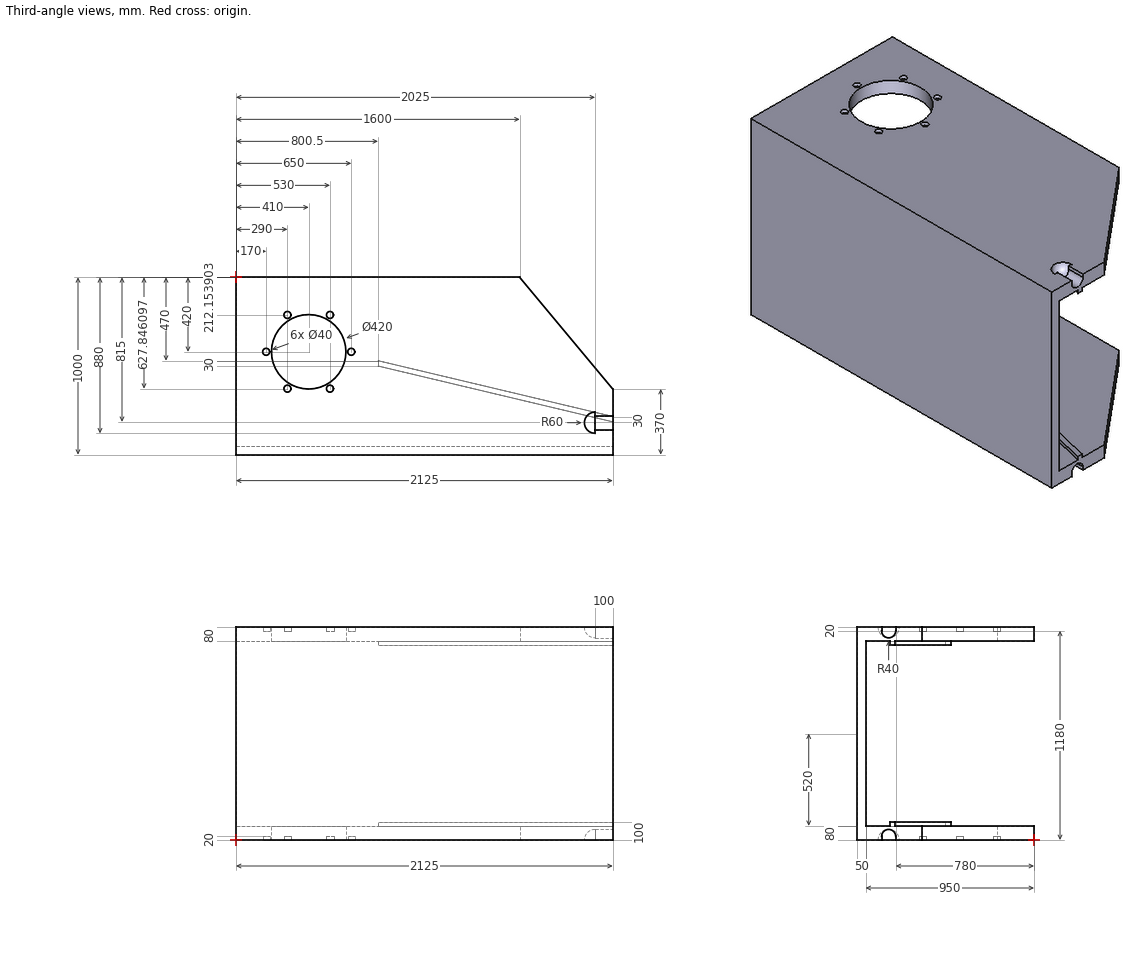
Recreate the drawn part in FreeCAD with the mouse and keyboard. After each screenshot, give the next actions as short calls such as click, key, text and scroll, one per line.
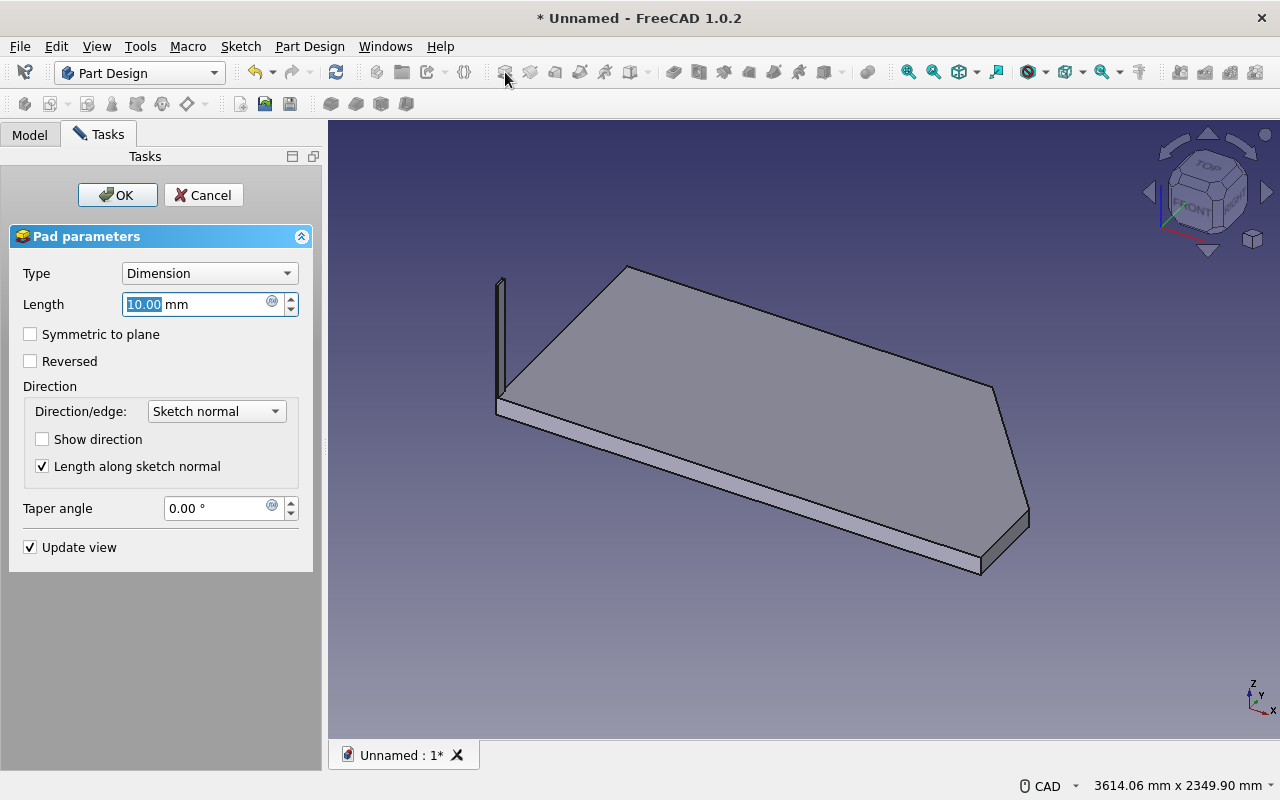
text(2125)
key(Tab)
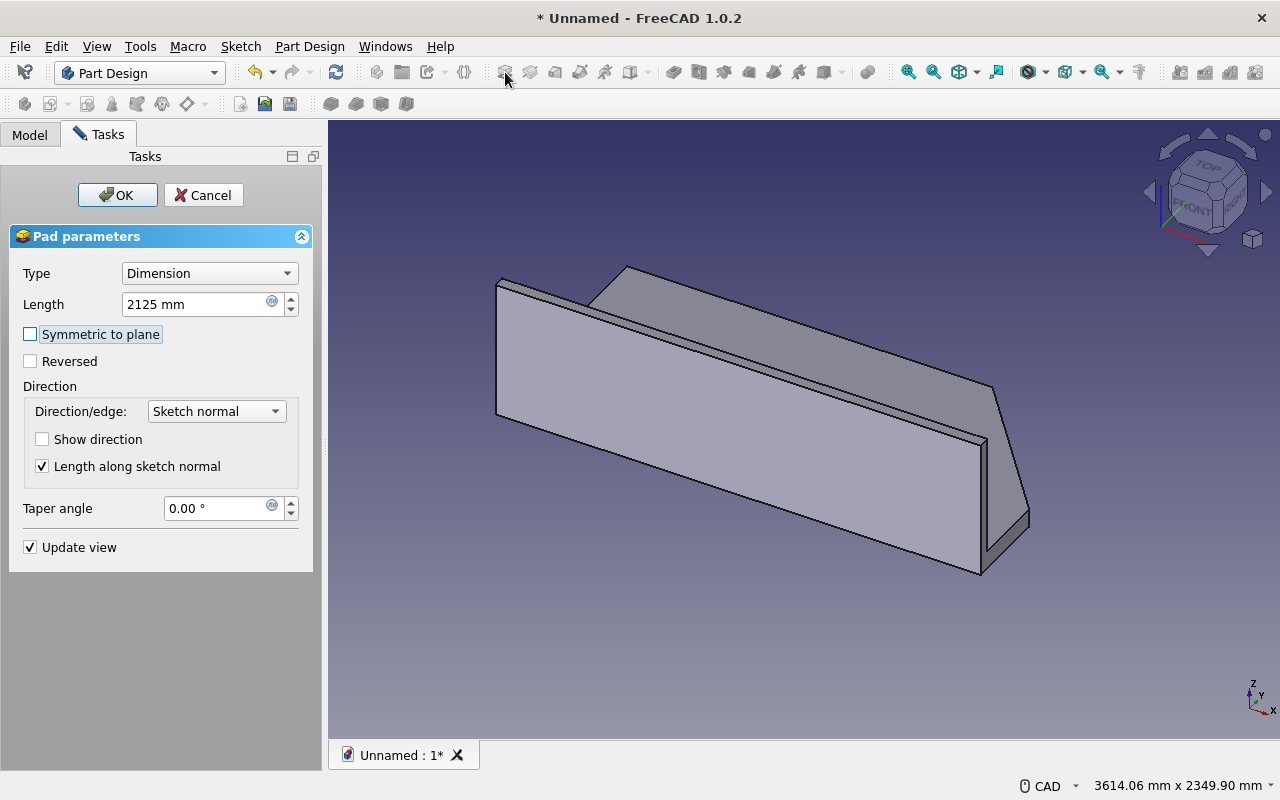
click(118, 195)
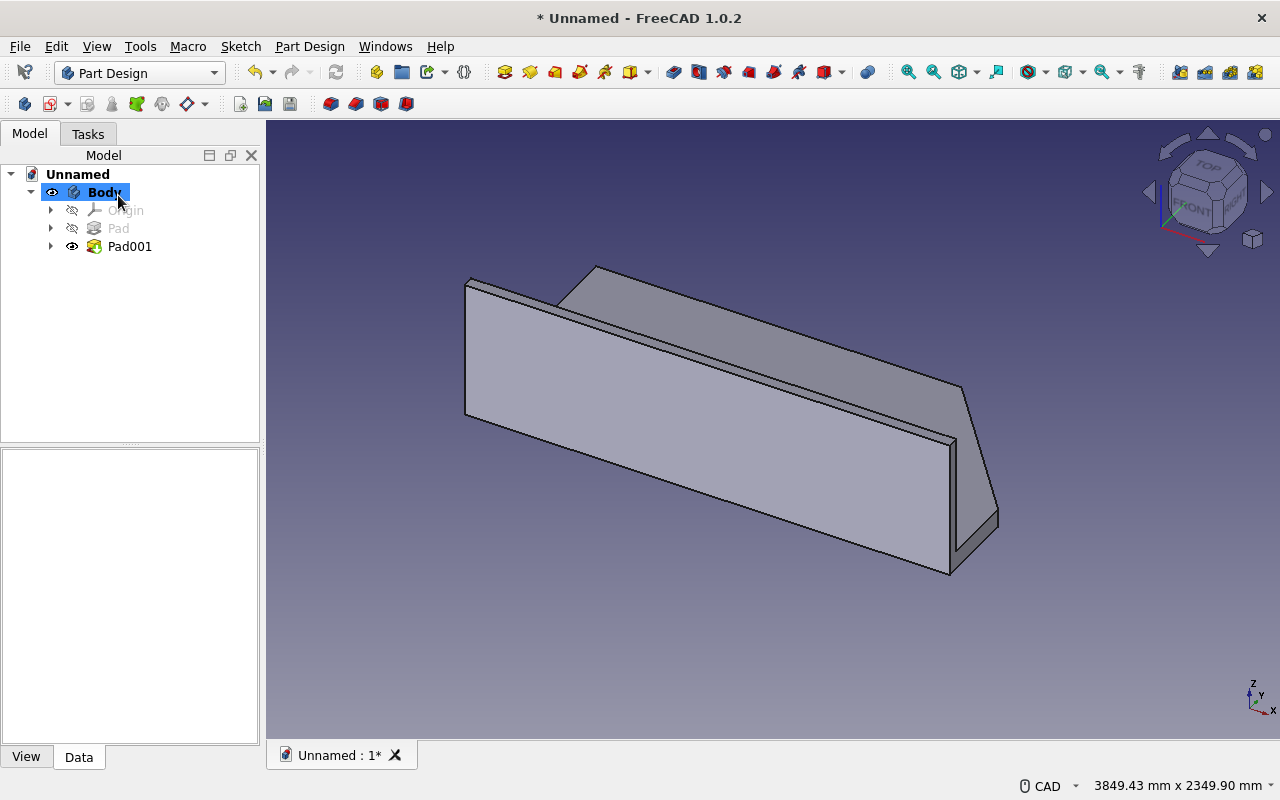
click(51, 210)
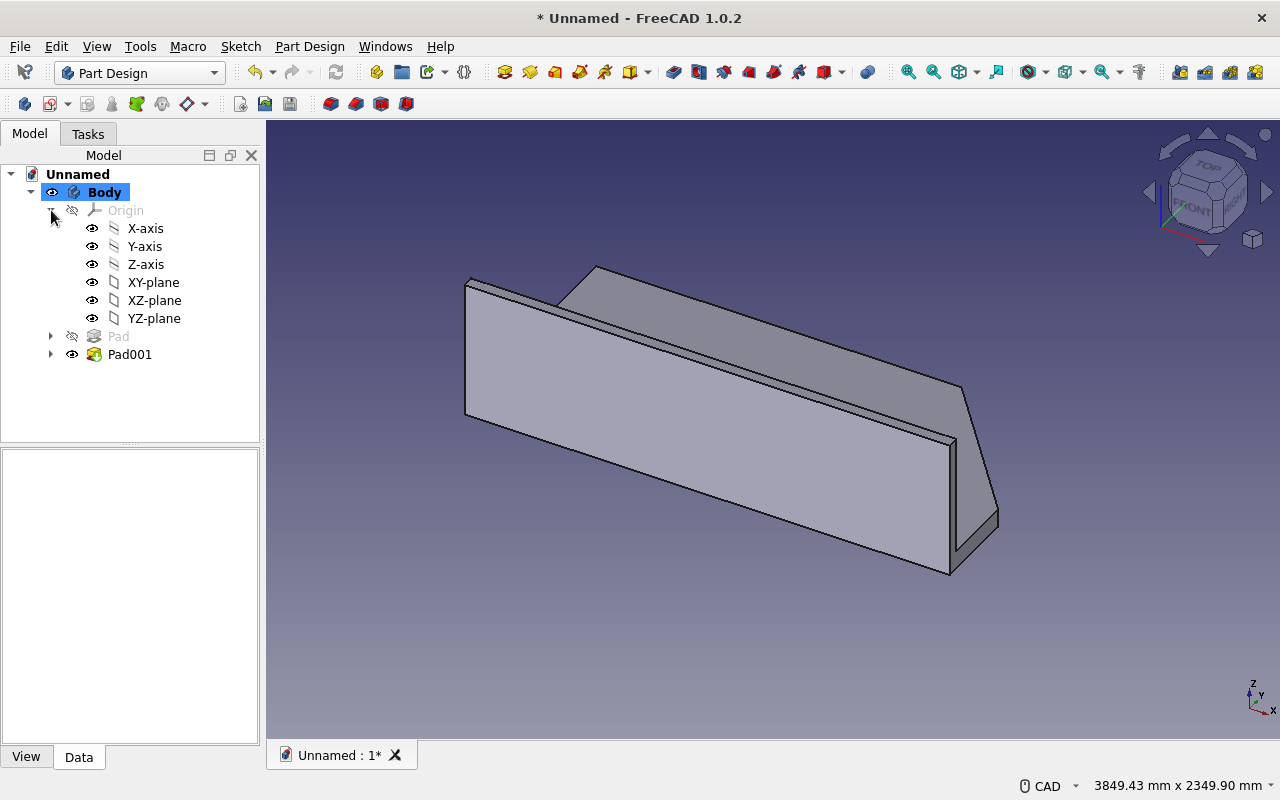
click(137, 282)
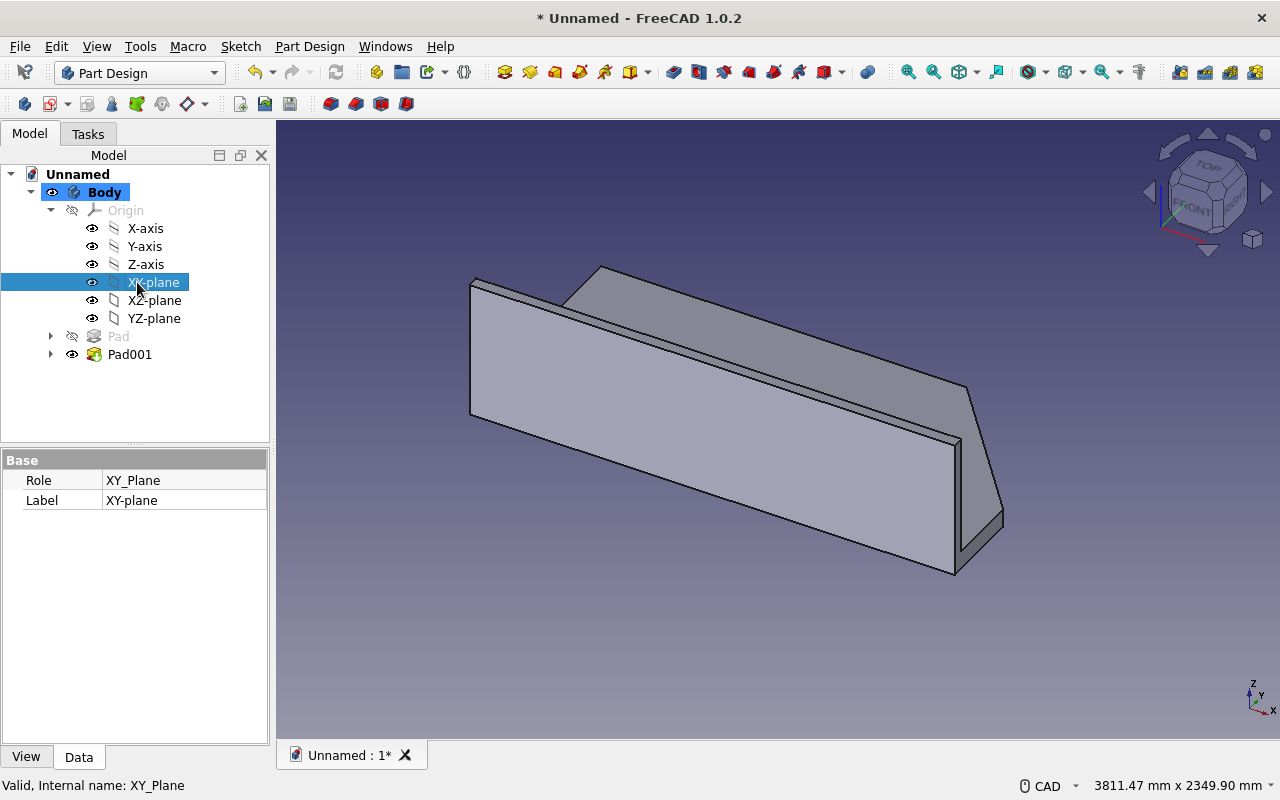
click(186, 104)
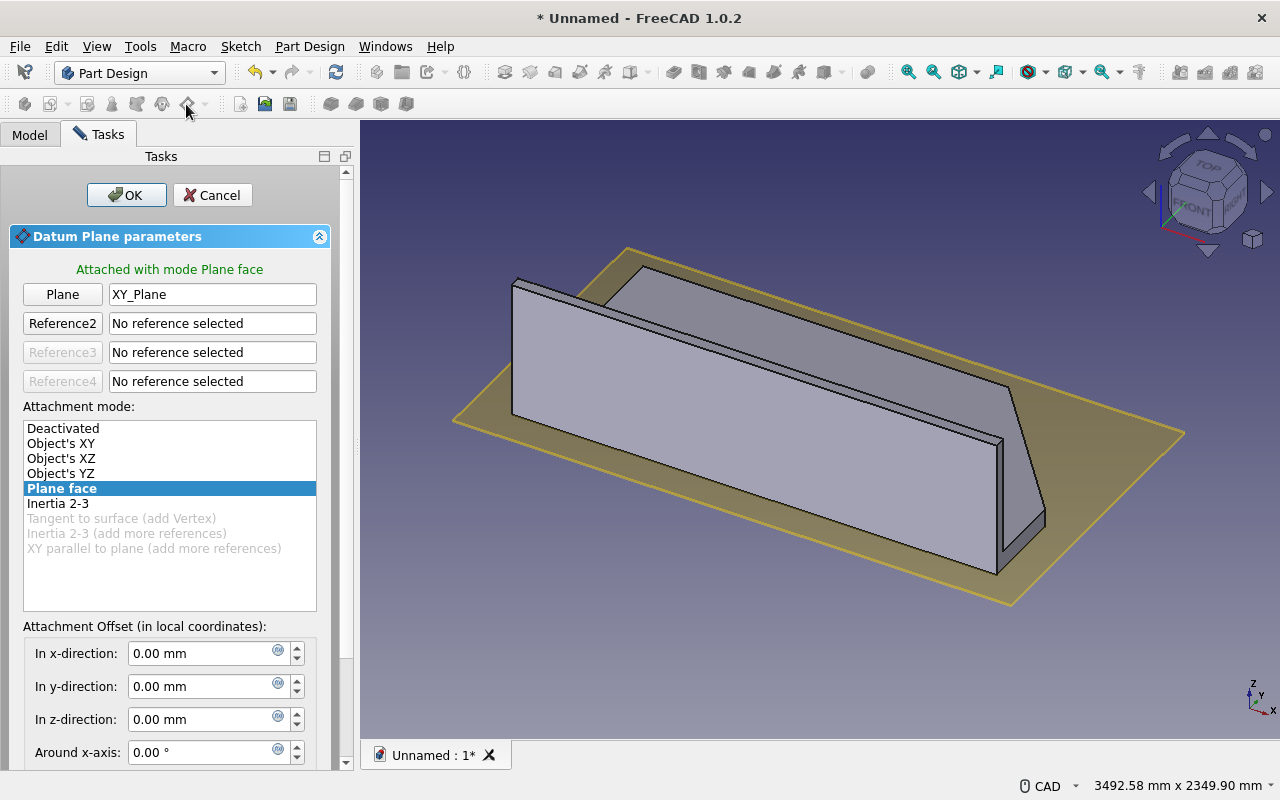
triple_click(210, 720)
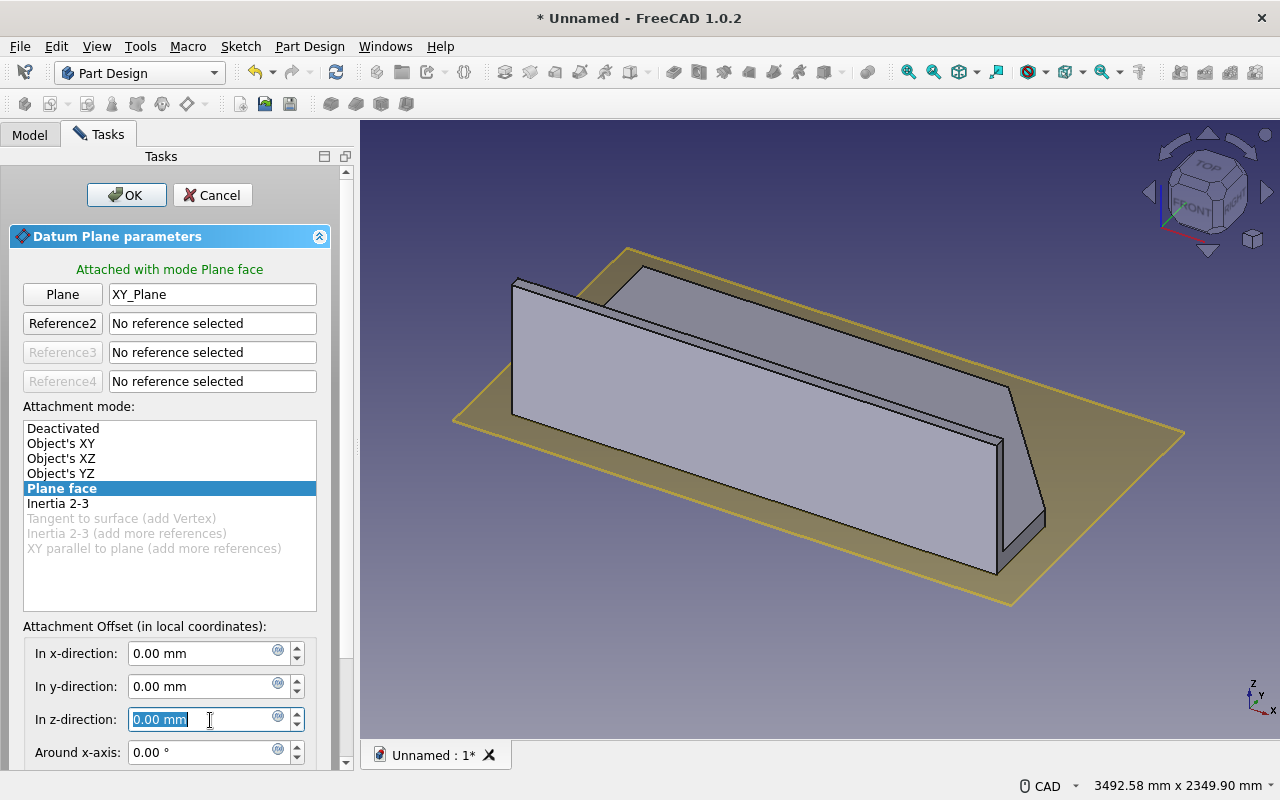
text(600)
key(Tab)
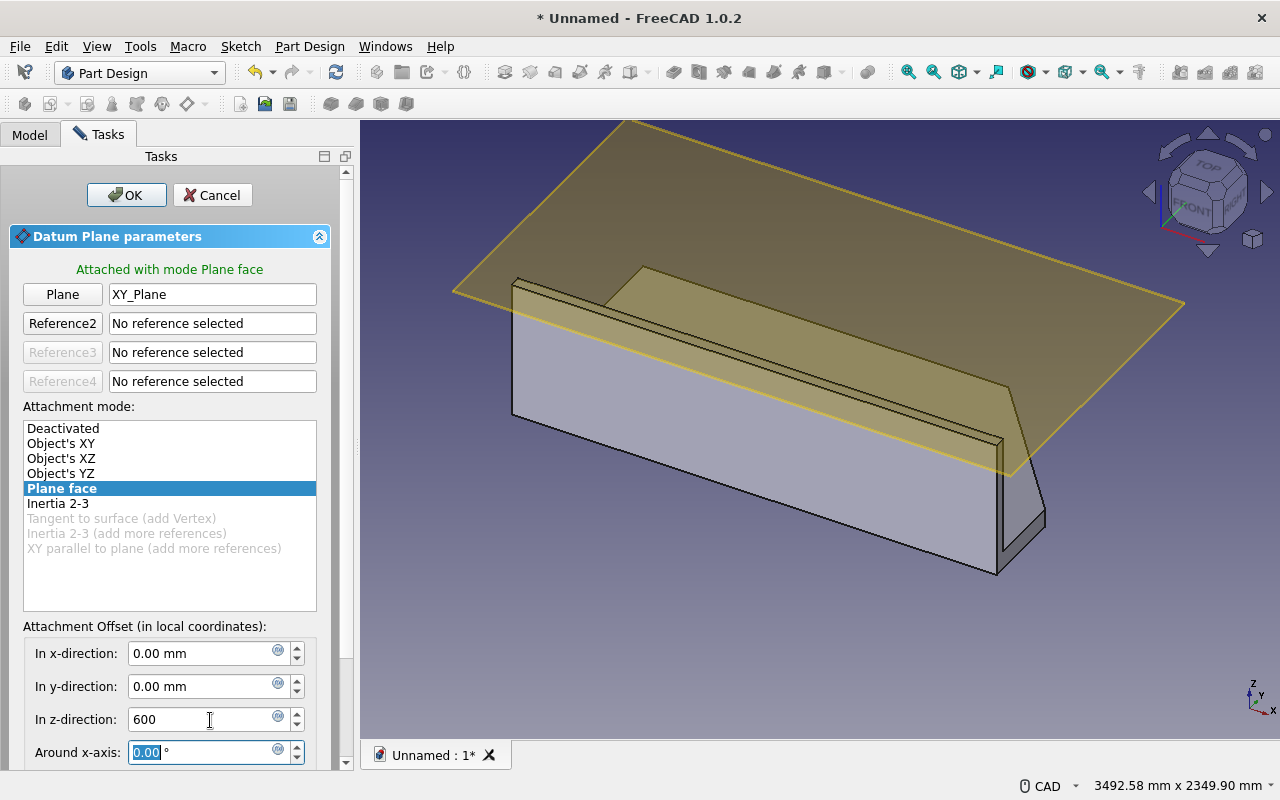
click(127, 195)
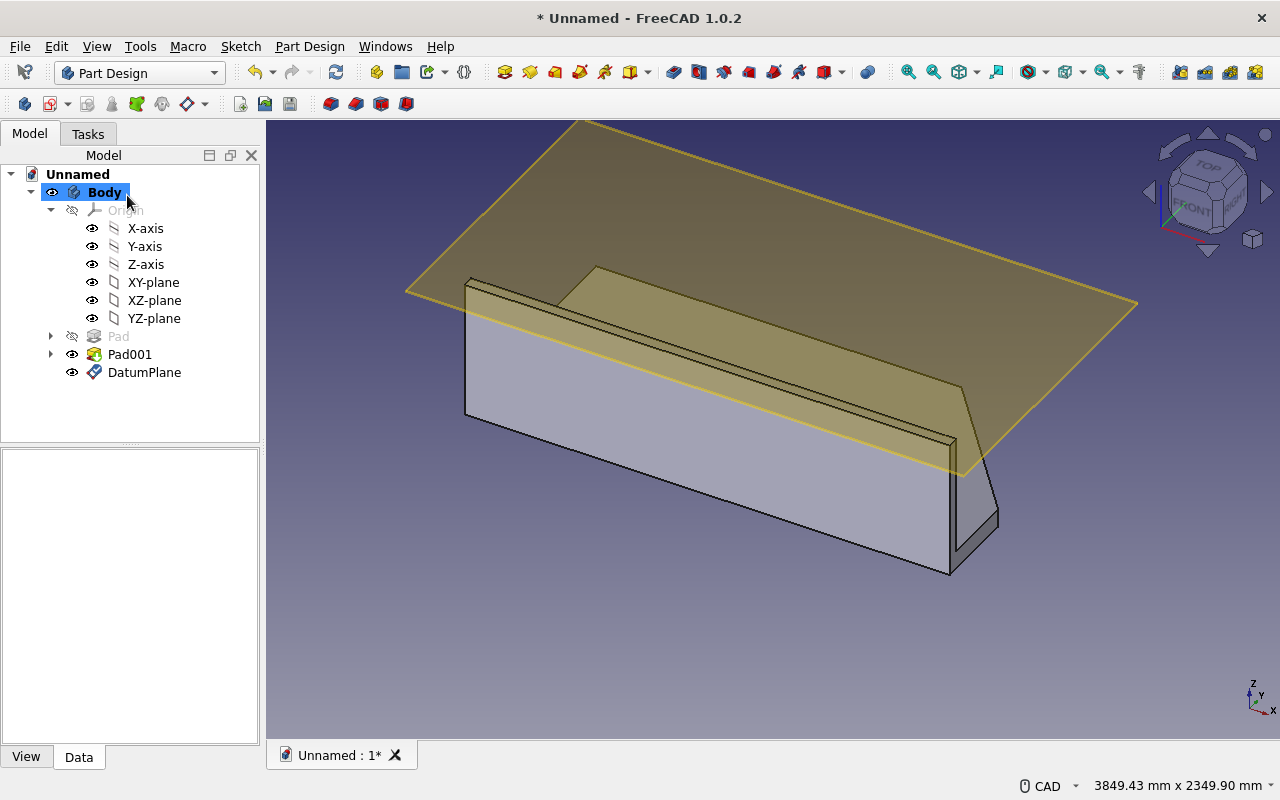
click(117, 354)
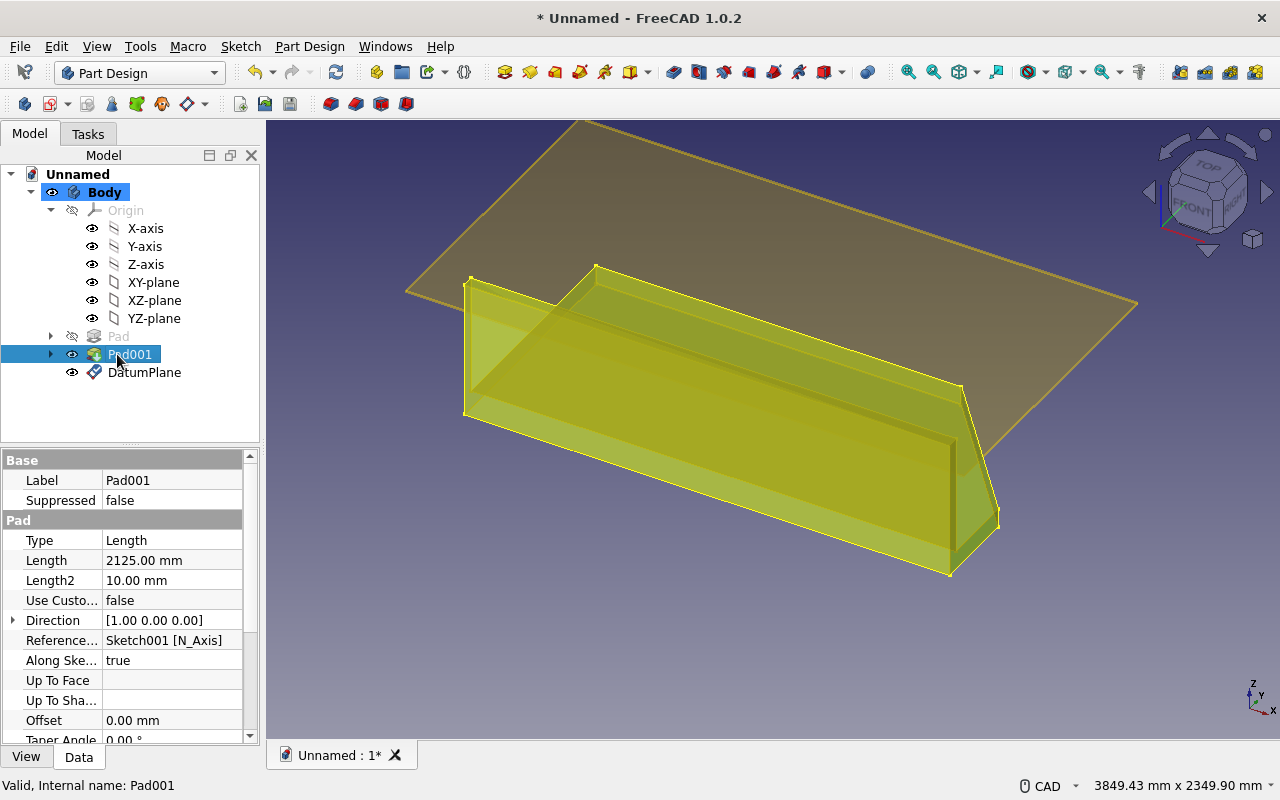
click(1180, 72)